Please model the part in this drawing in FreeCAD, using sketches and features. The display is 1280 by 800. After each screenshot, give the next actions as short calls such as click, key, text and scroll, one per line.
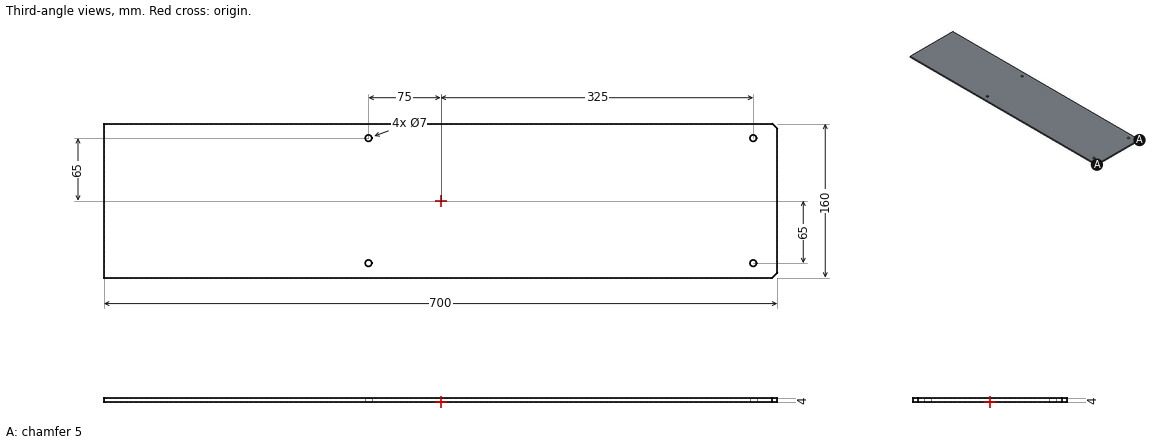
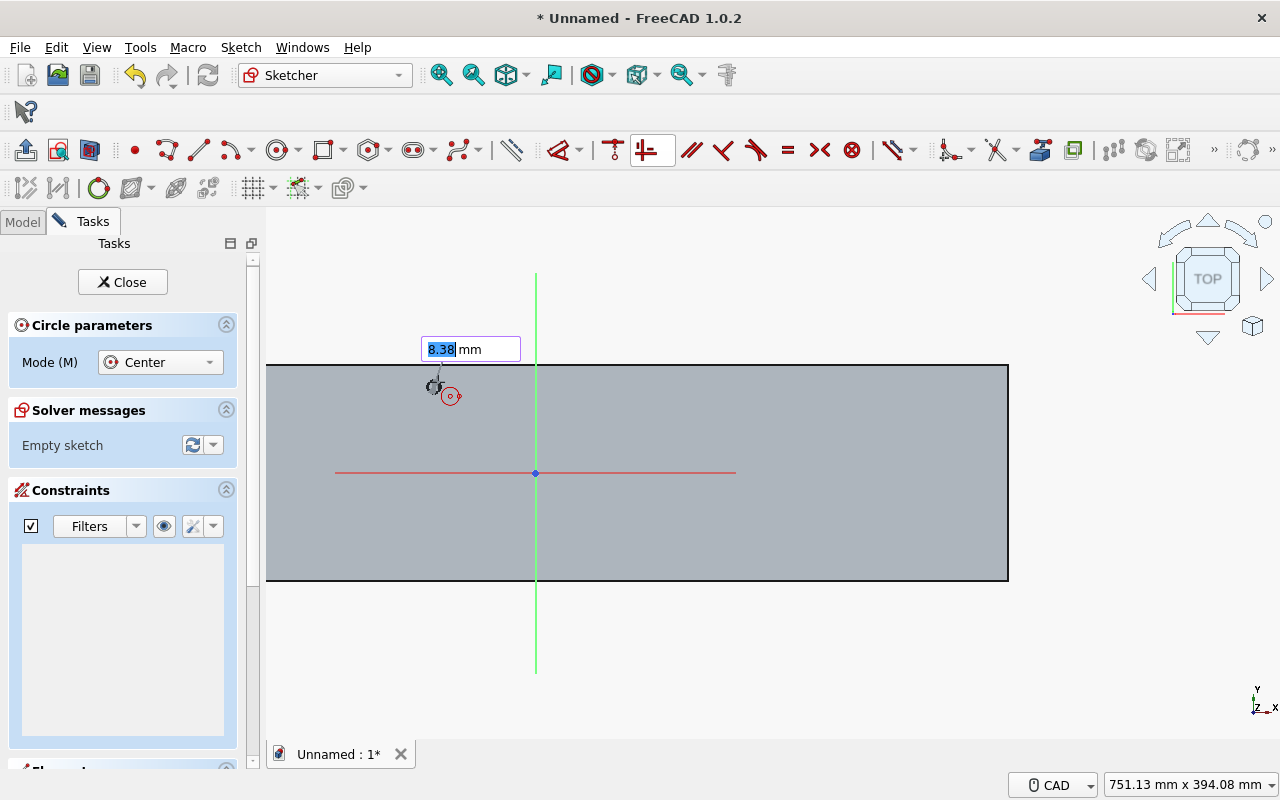
text(7)
key(Return)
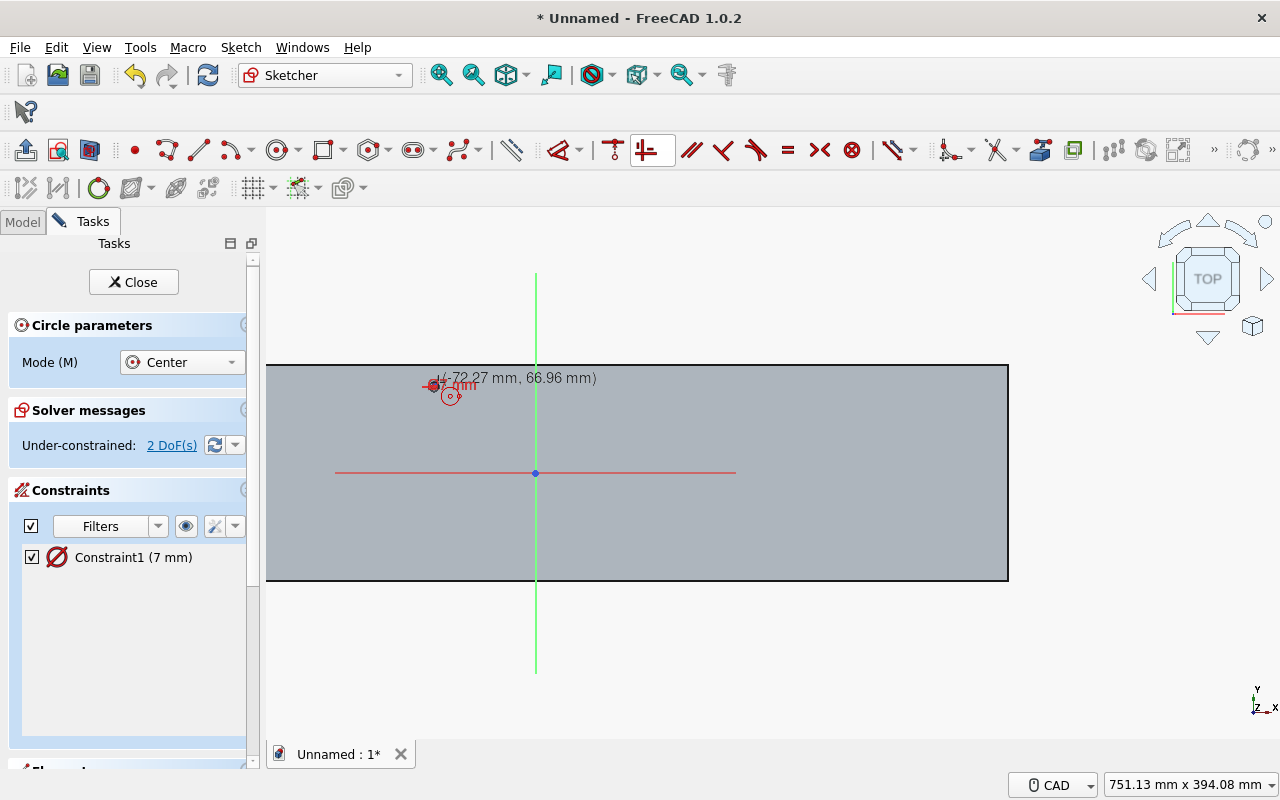
scroll(974, 386, up, 8)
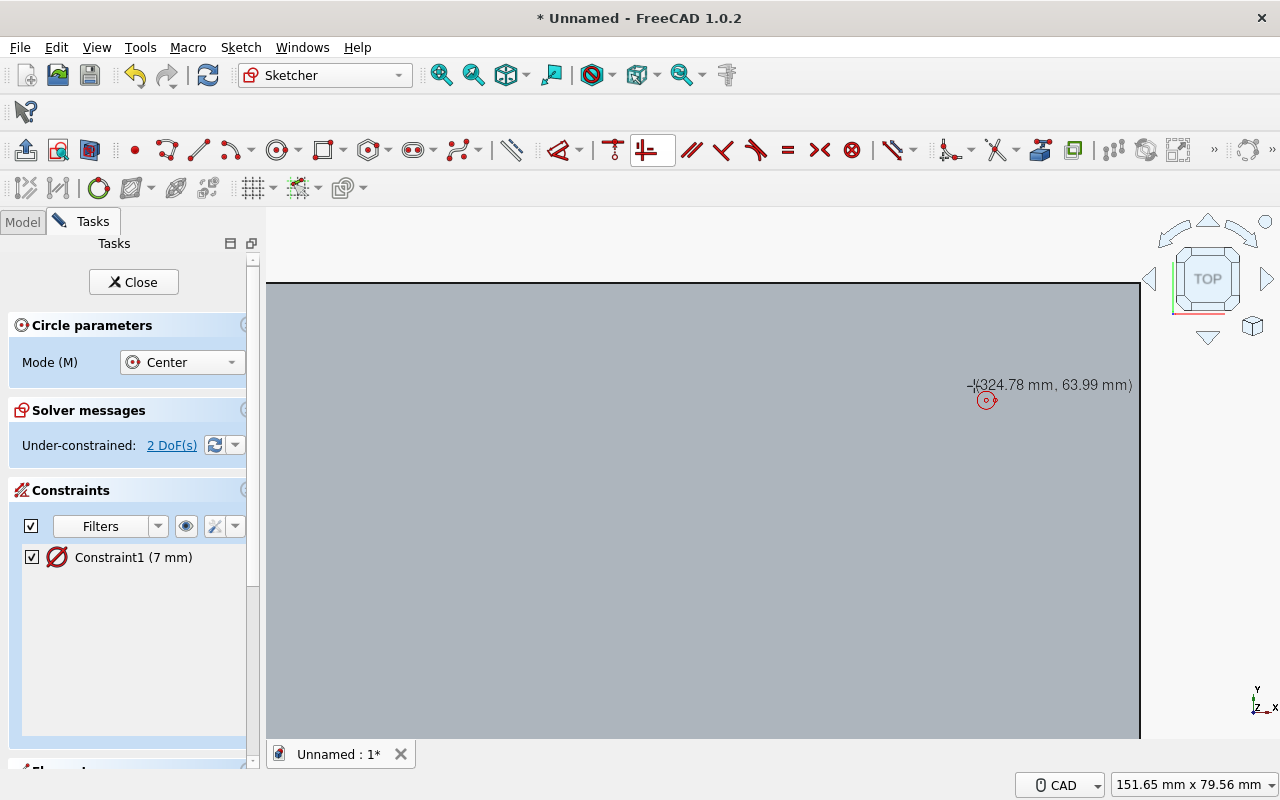
scroll(975, 386, down, 8)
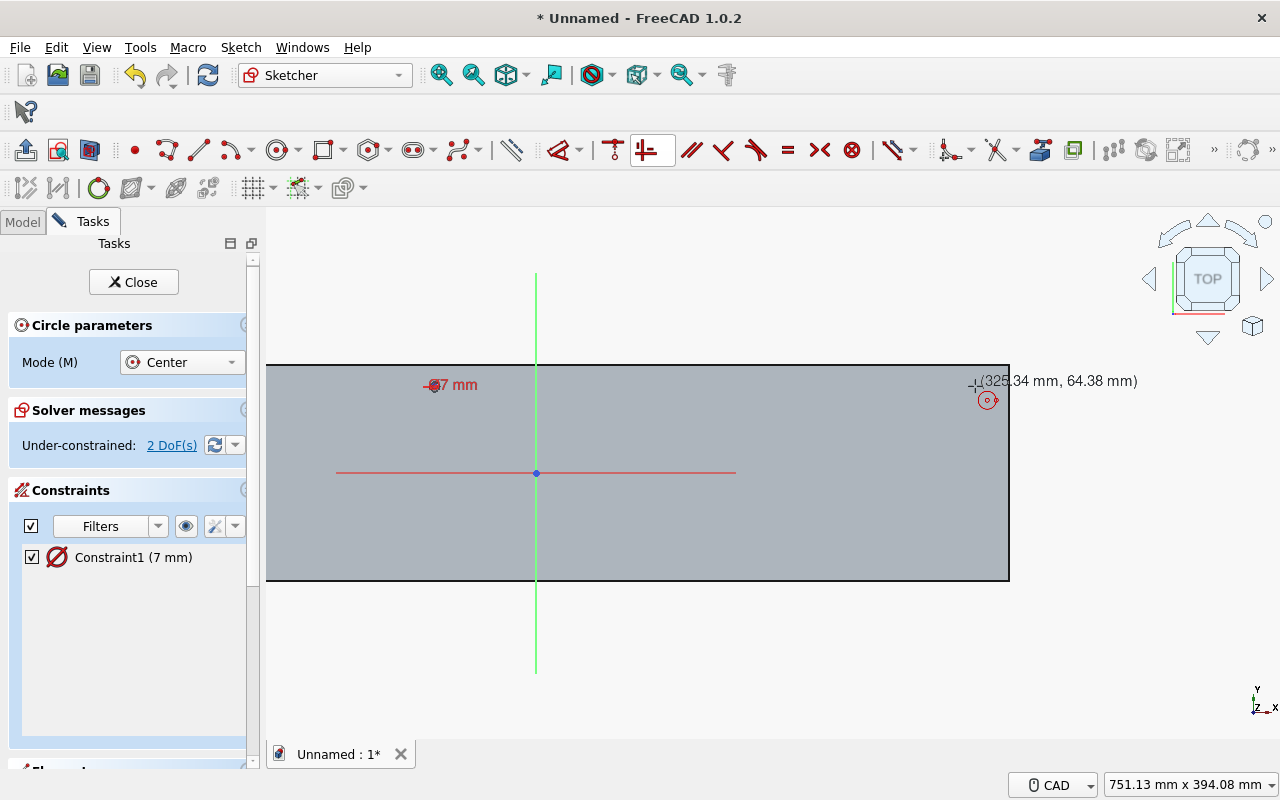
click(975, 386)
move(978, 382)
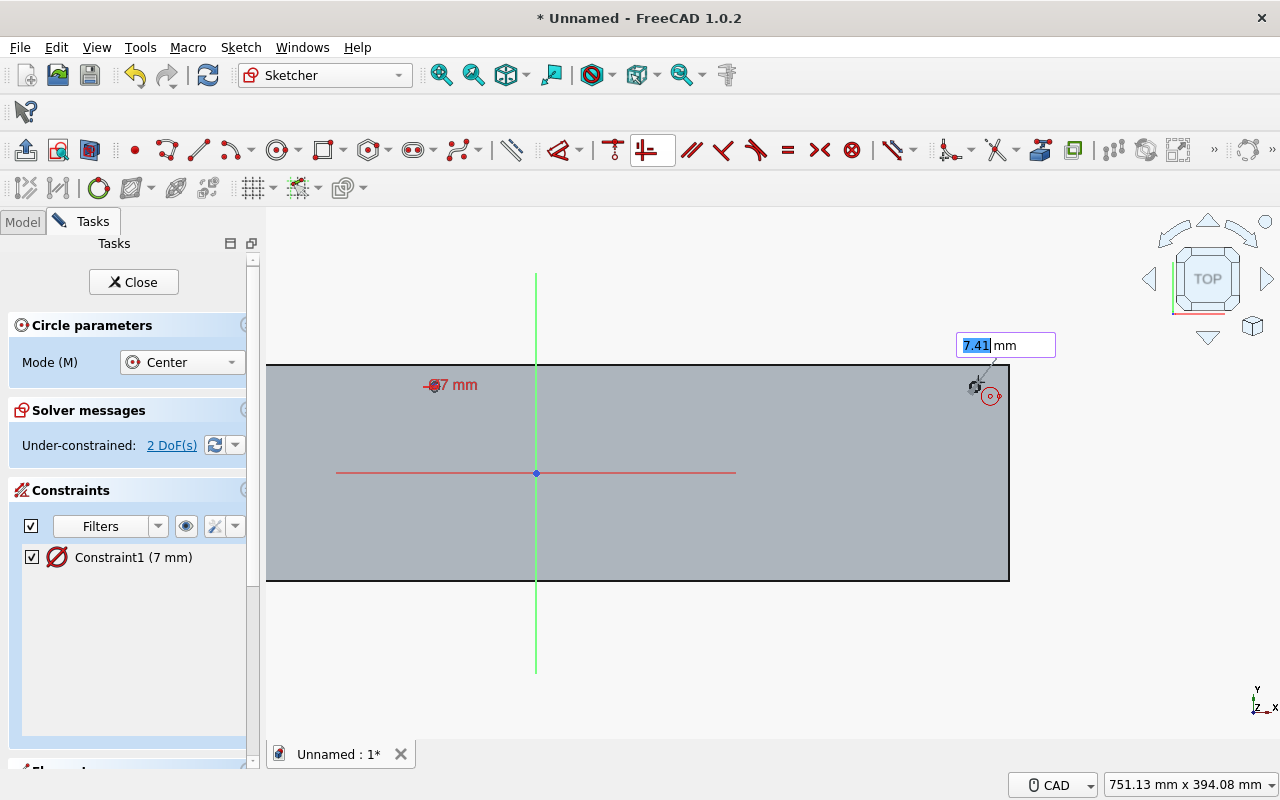
text(7)
key(Return)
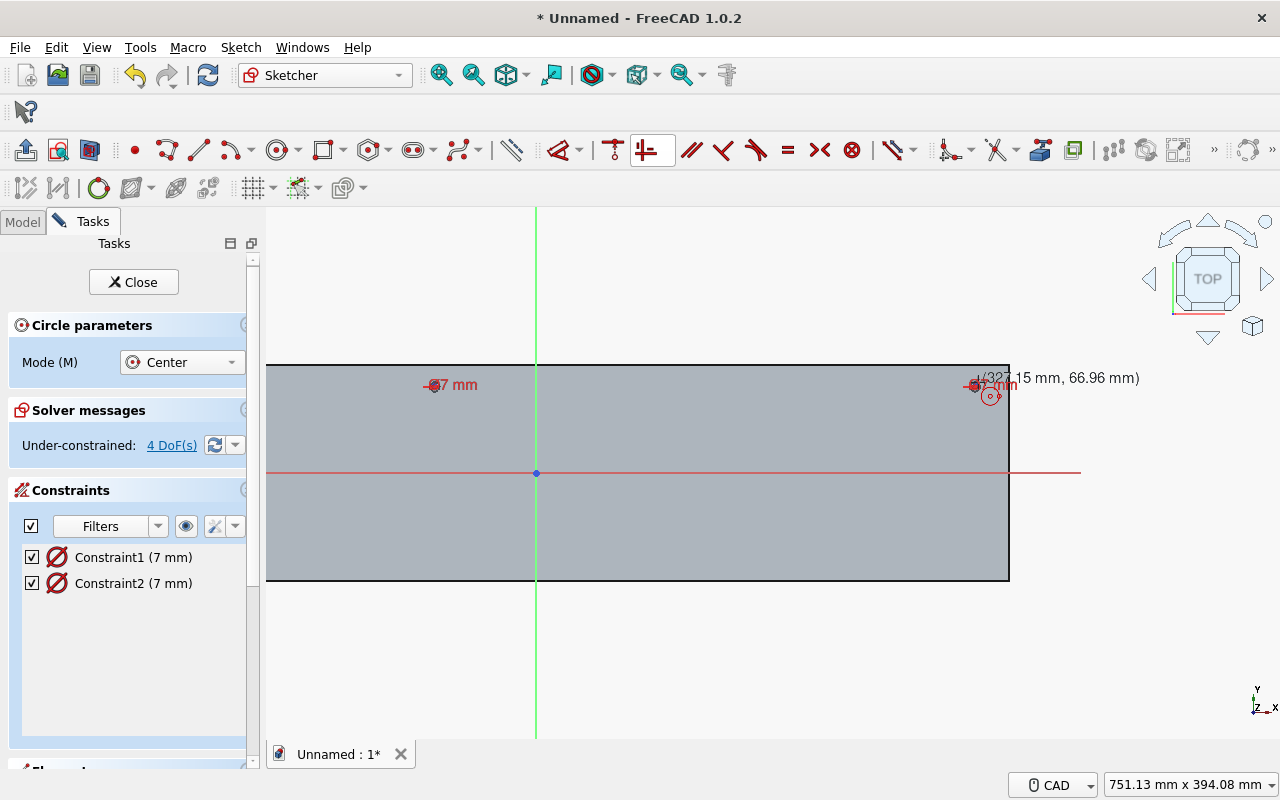
scroll(975, 561, up, 8)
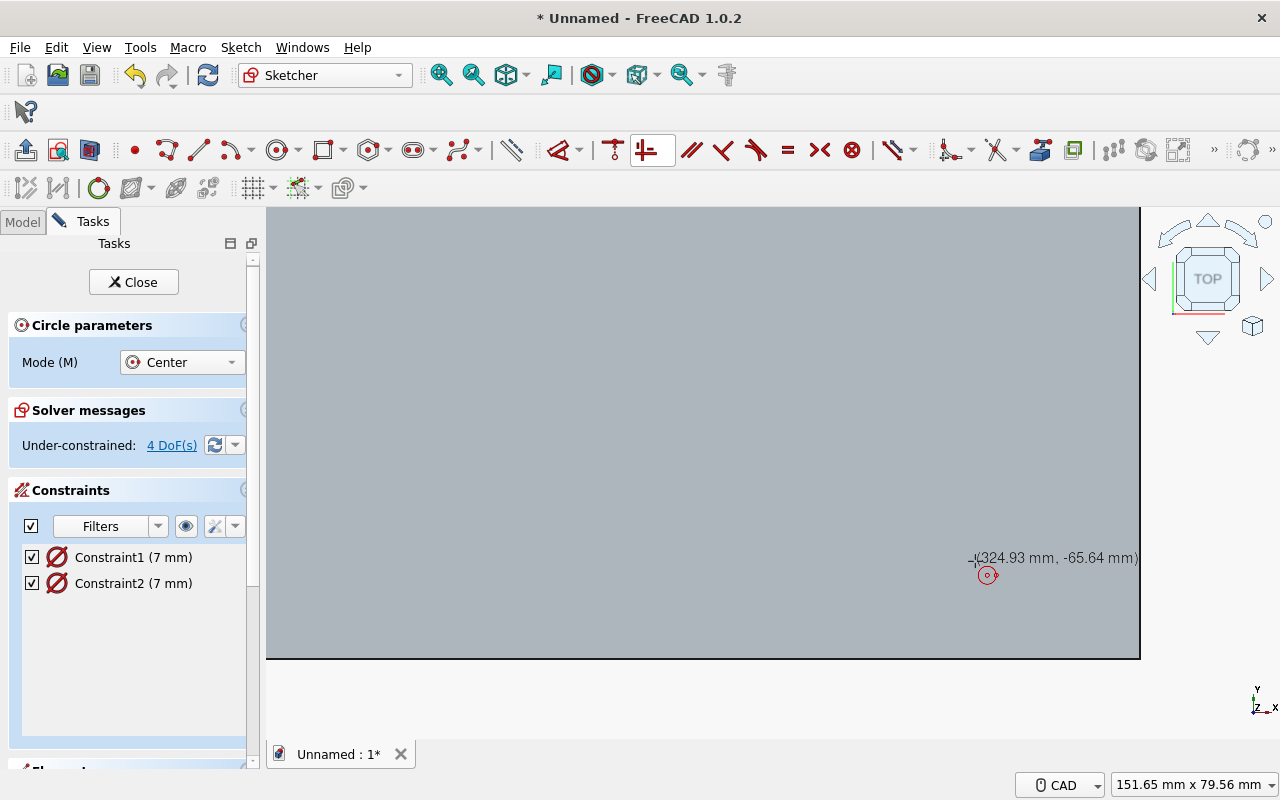
scroll(975, 561, down, 8)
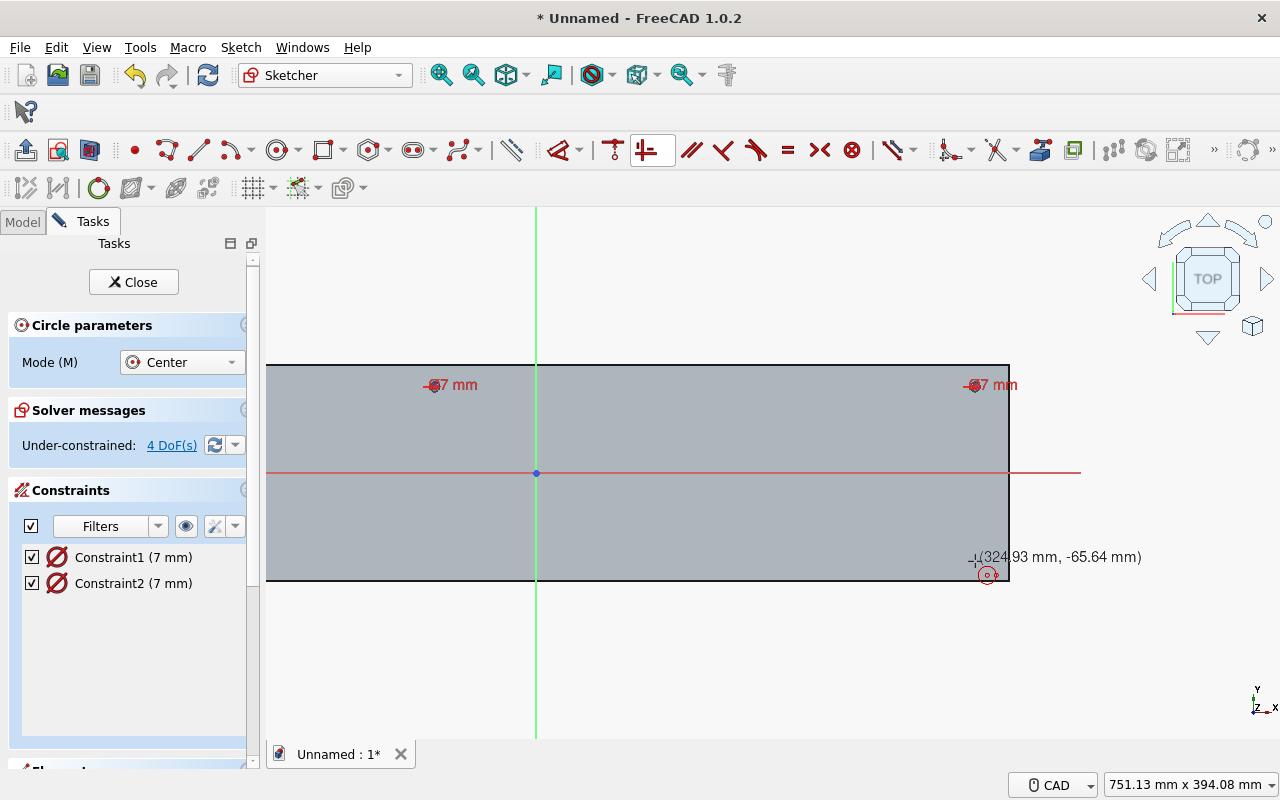
click(975, 561)
move(978, 558)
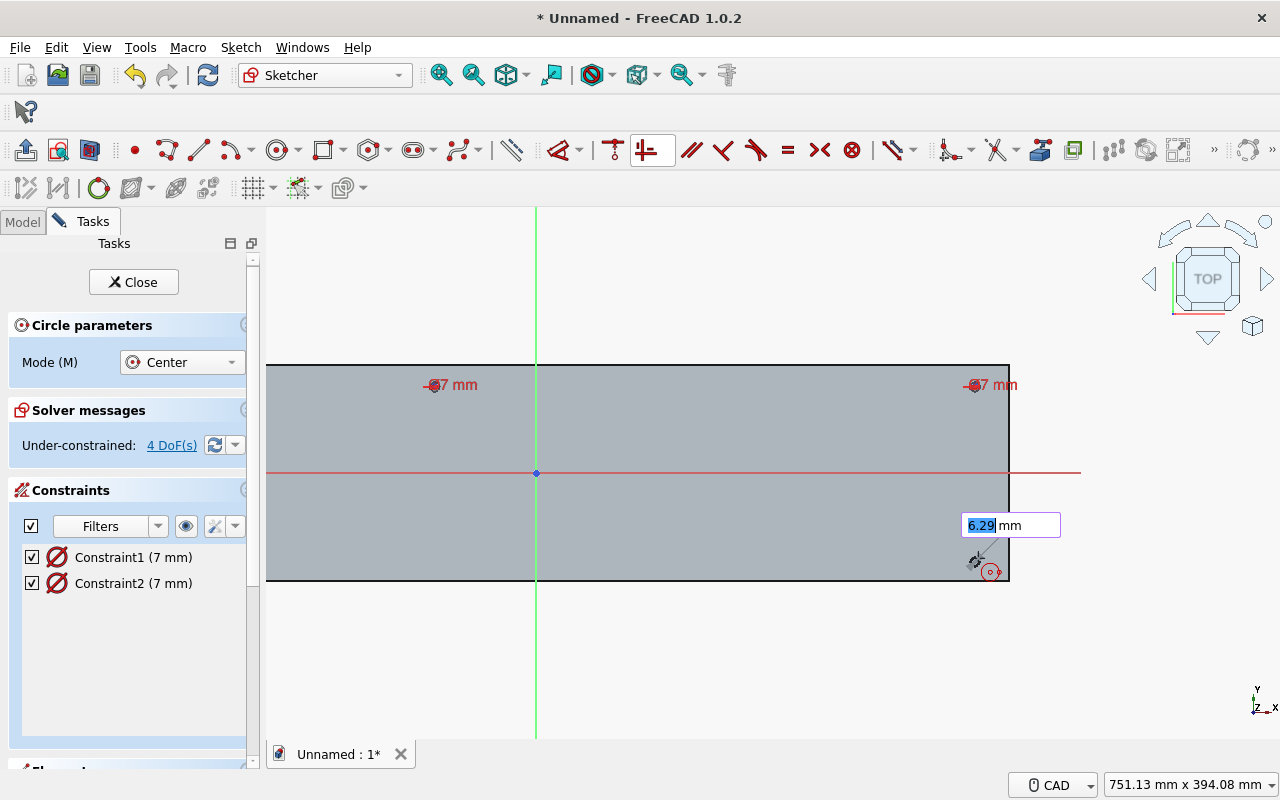
text(7)
key(Return)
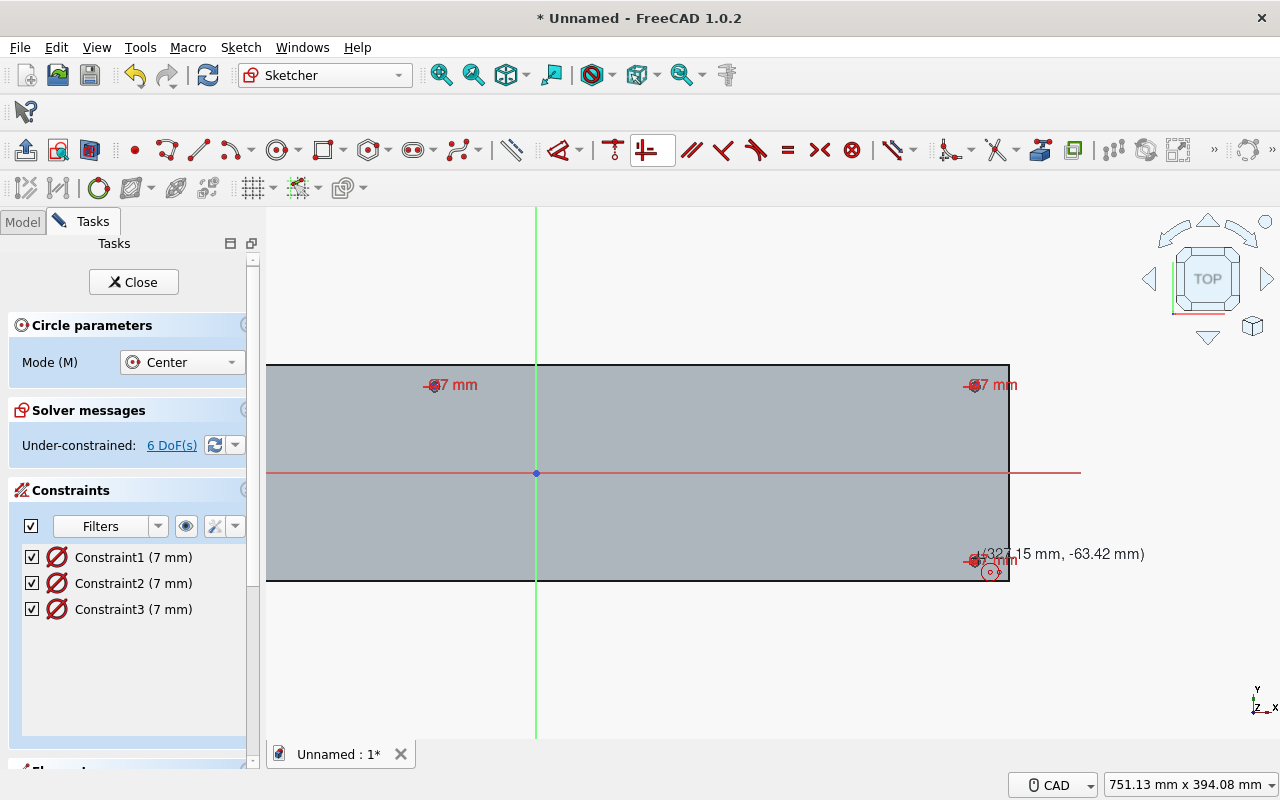
scroll(435, 561, up, 8)